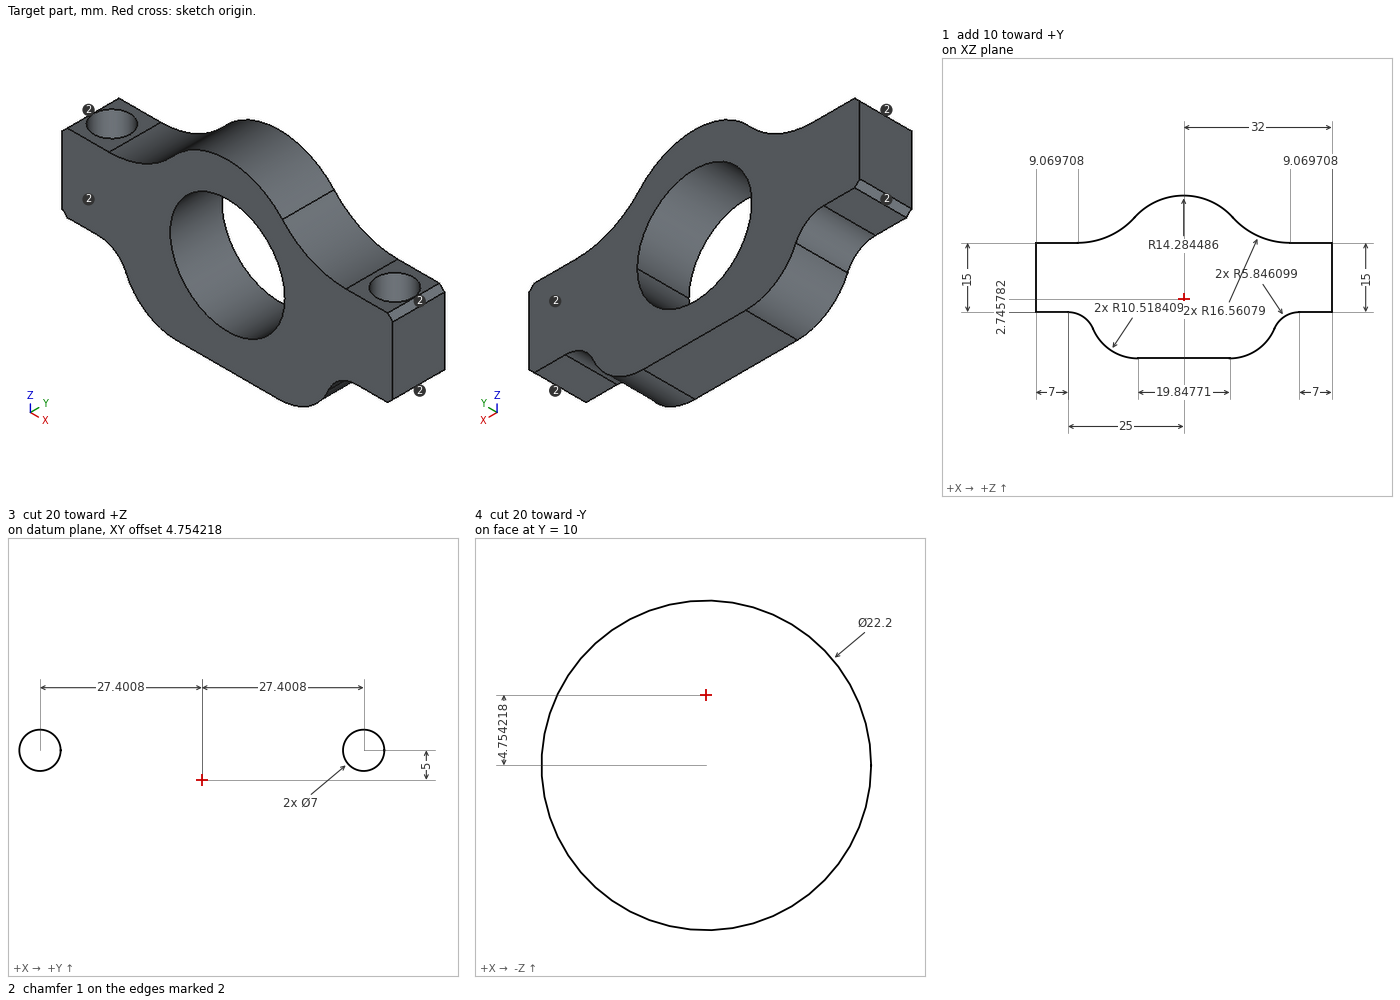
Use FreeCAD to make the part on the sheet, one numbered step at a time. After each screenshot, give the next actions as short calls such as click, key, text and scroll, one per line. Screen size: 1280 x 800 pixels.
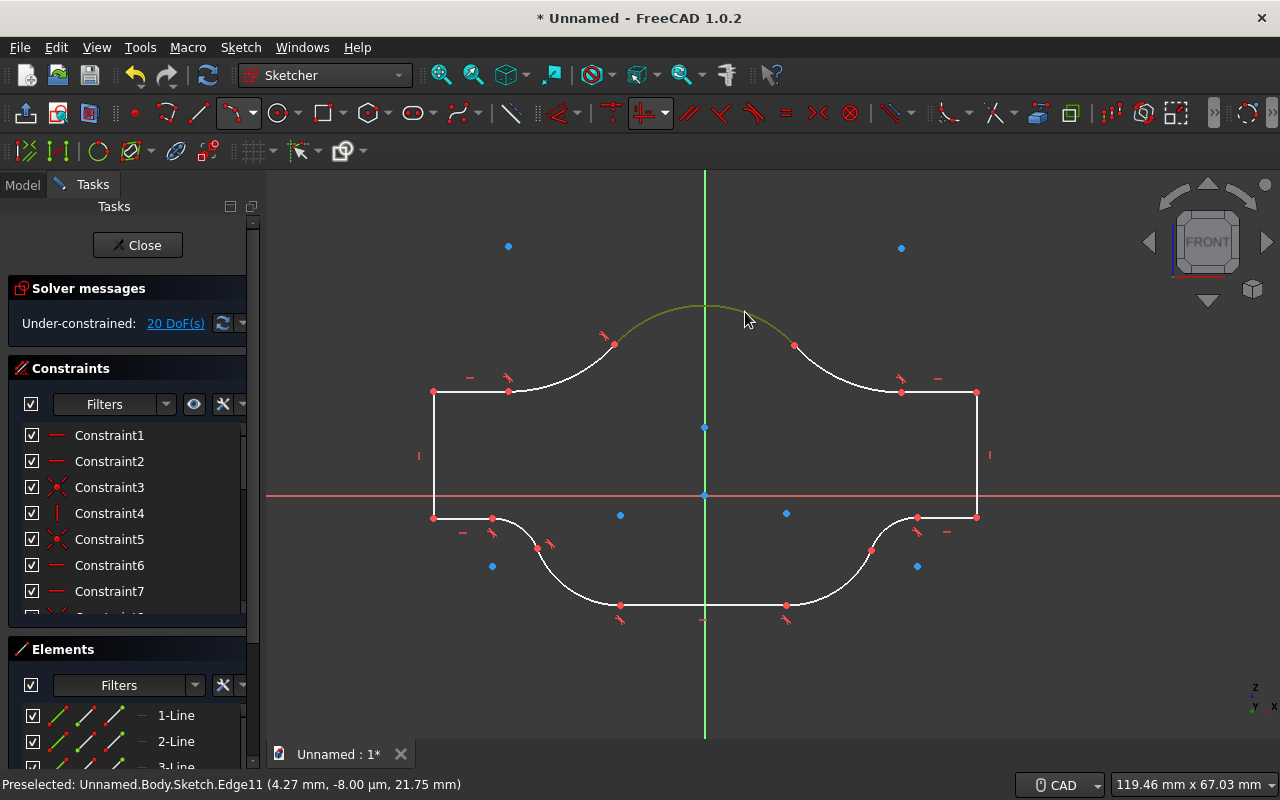
click(822, 369)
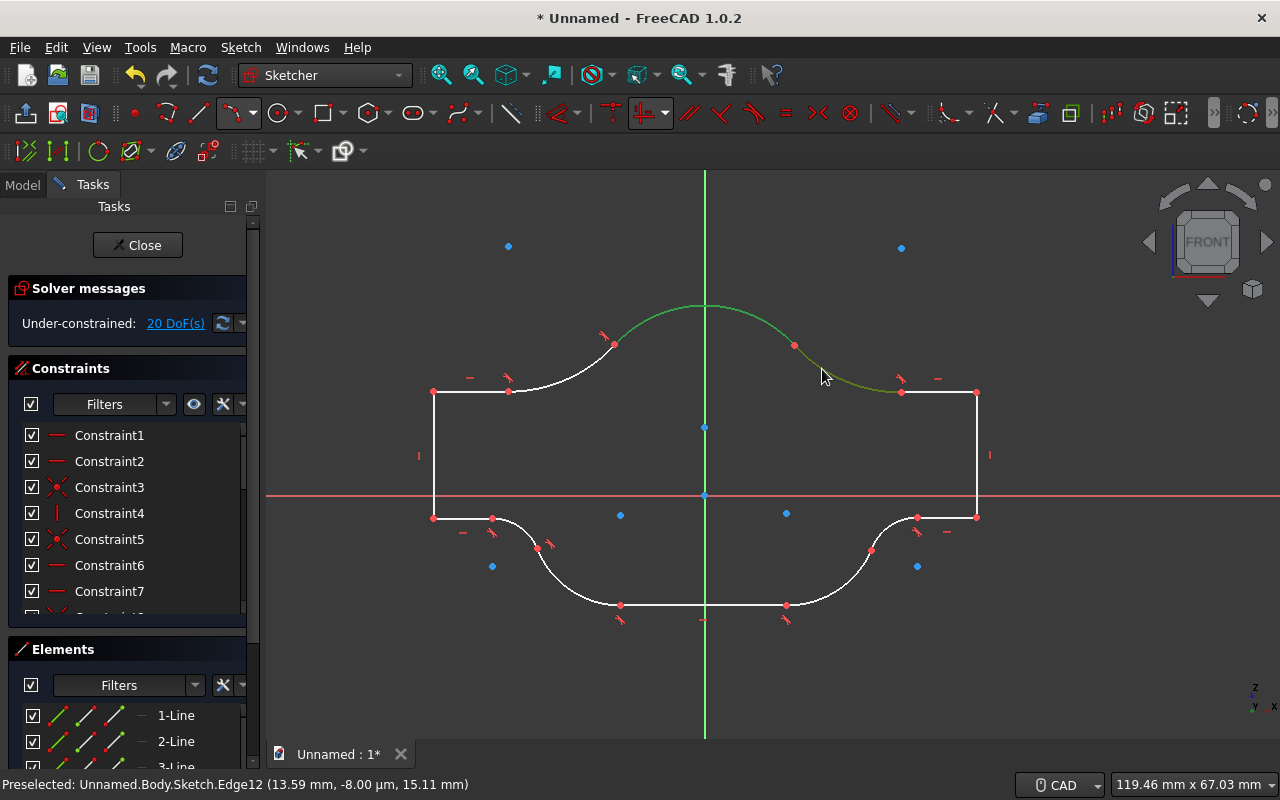
click(754, 114)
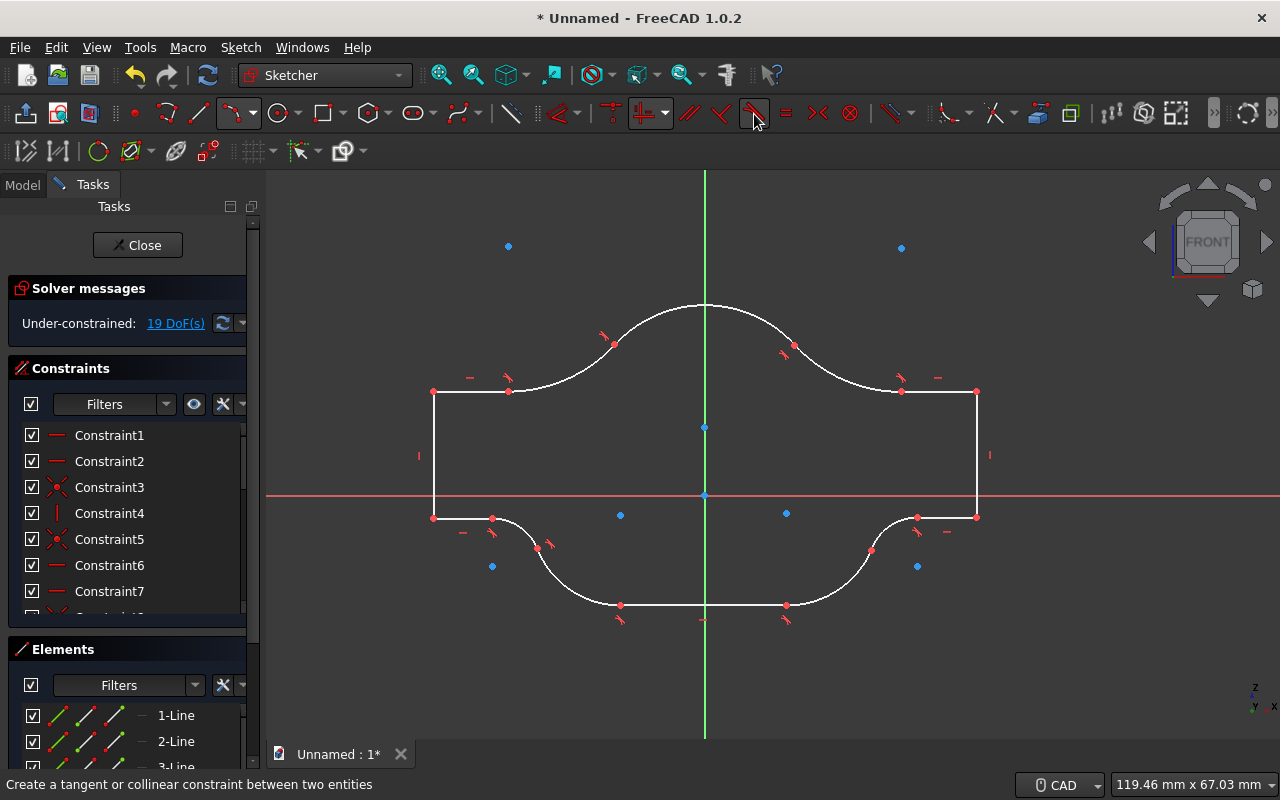
click(900, 521)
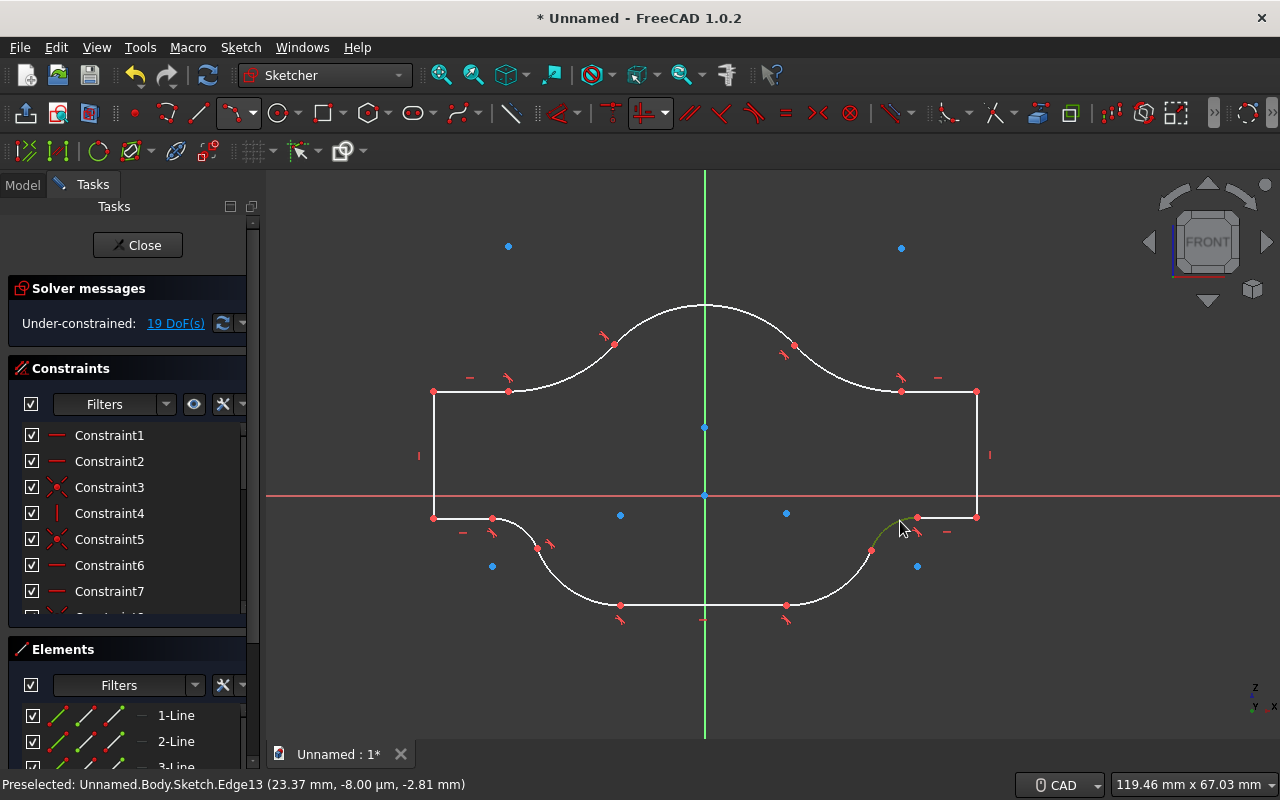
click(818, 600)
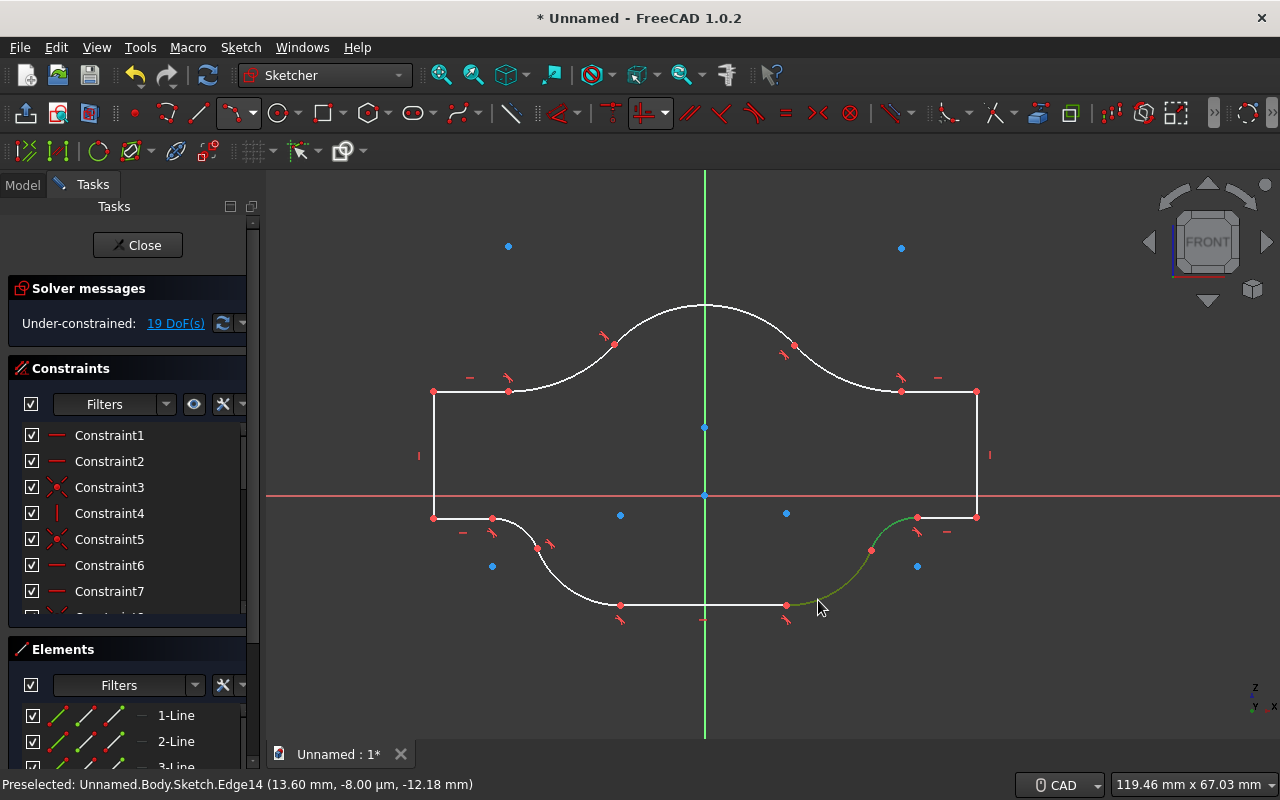
click(754, 114)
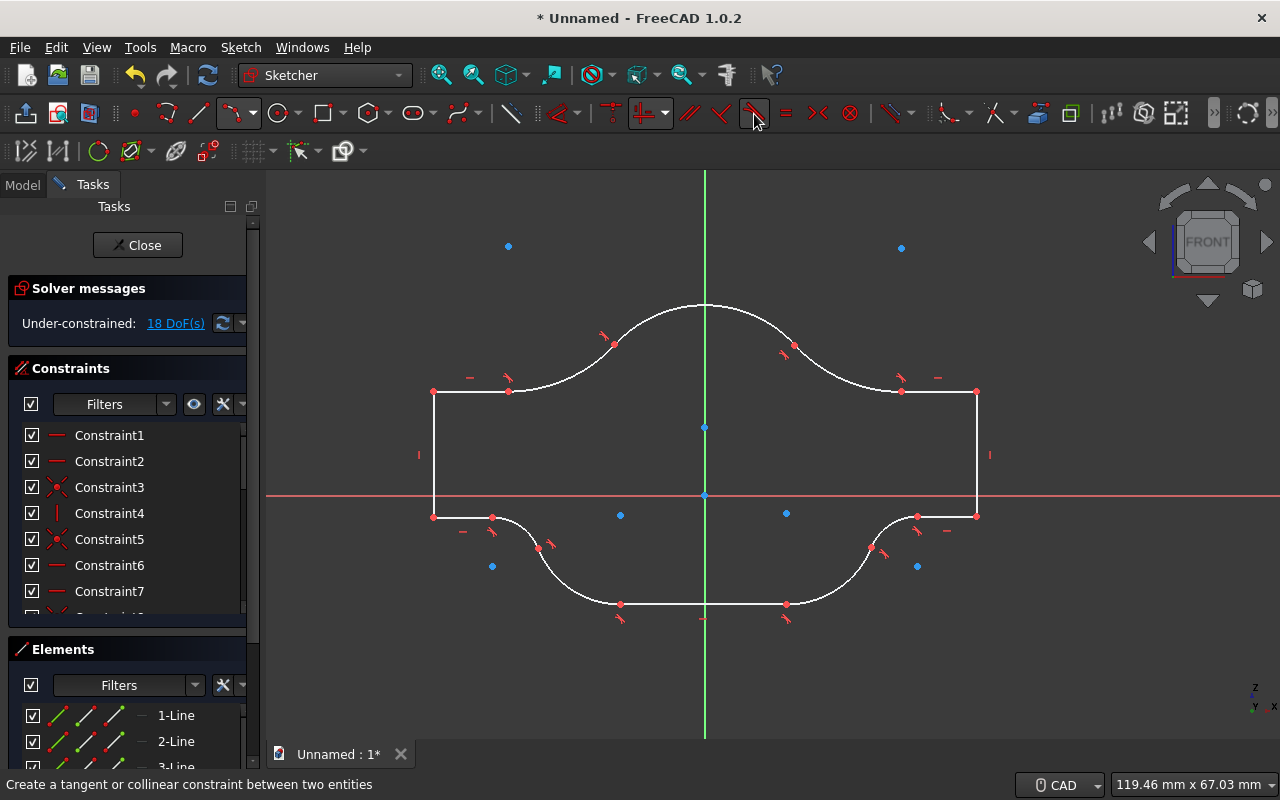
click(544, 387)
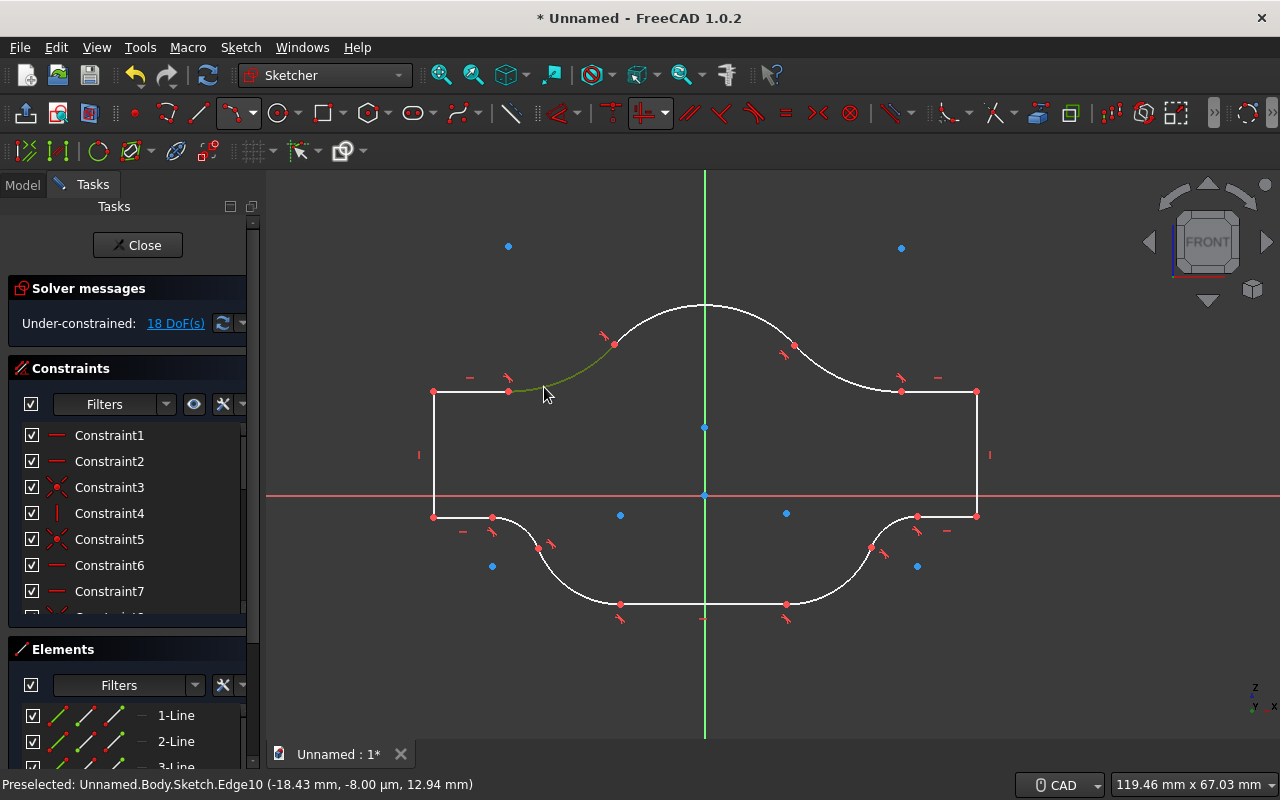
click(822, 368)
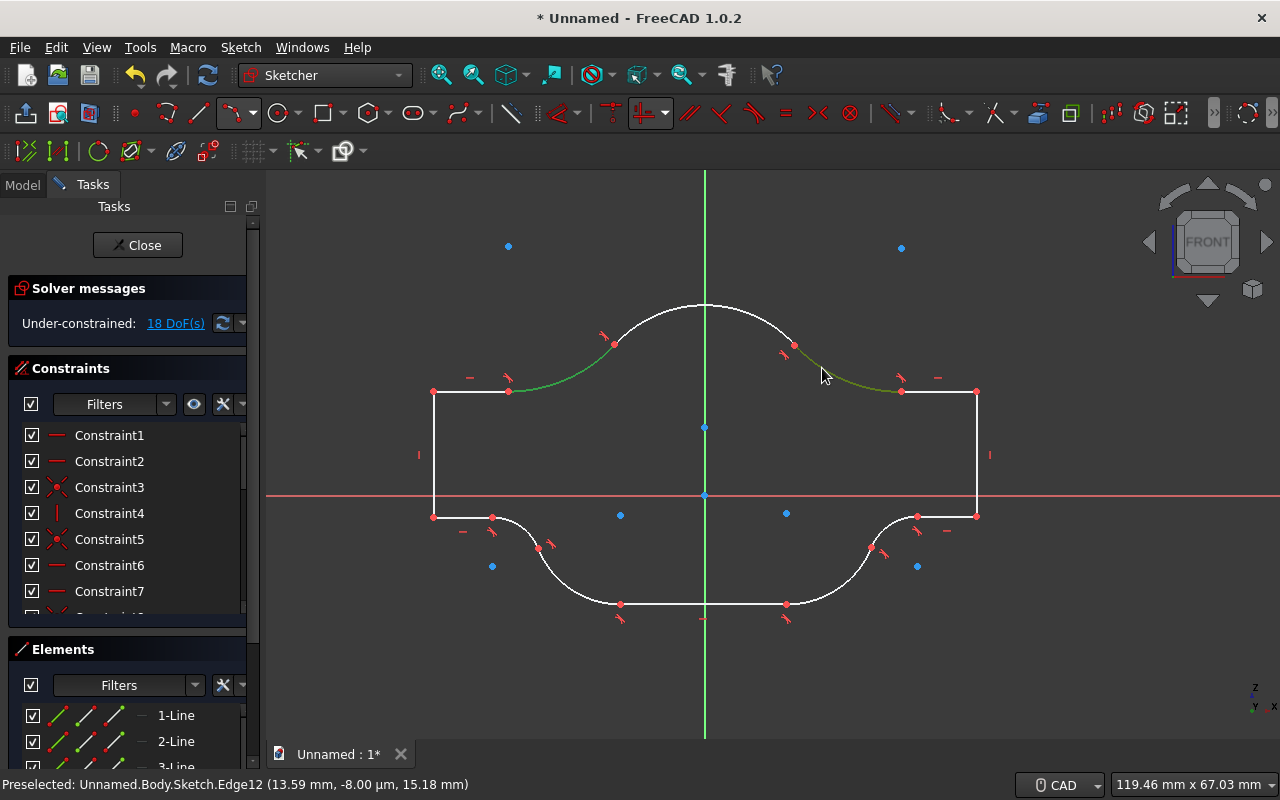
click(786, 114)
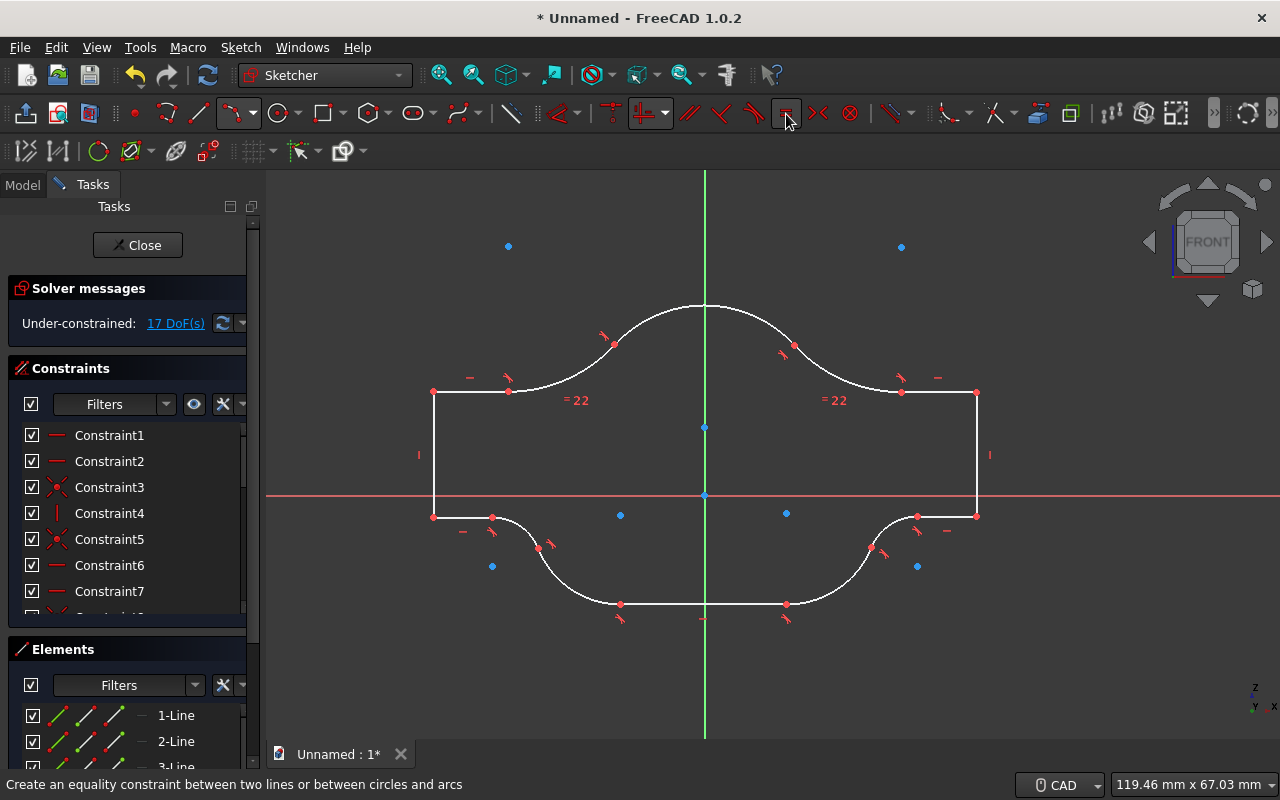
click(529, 534)